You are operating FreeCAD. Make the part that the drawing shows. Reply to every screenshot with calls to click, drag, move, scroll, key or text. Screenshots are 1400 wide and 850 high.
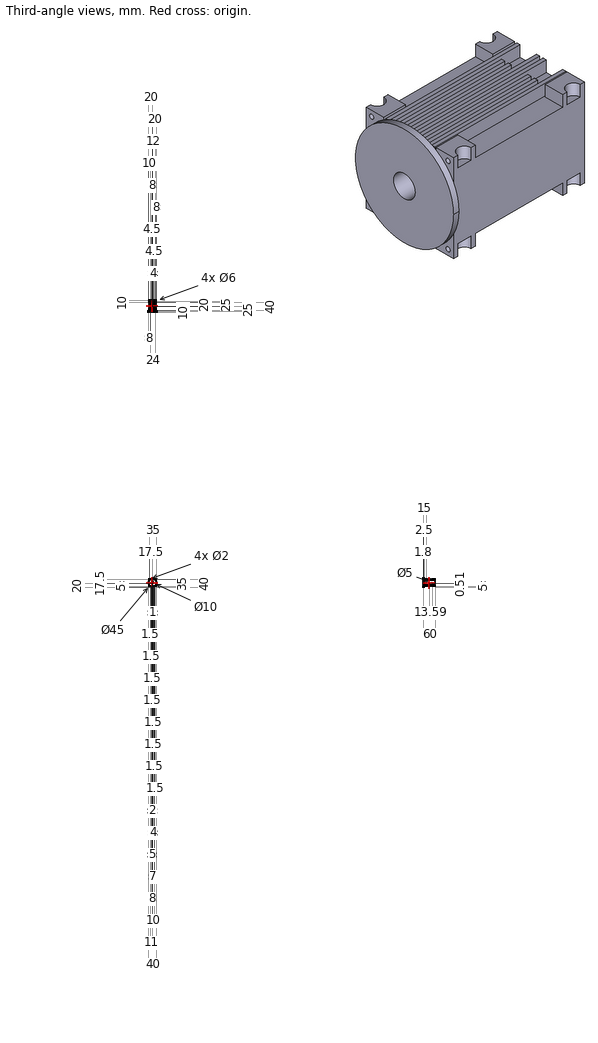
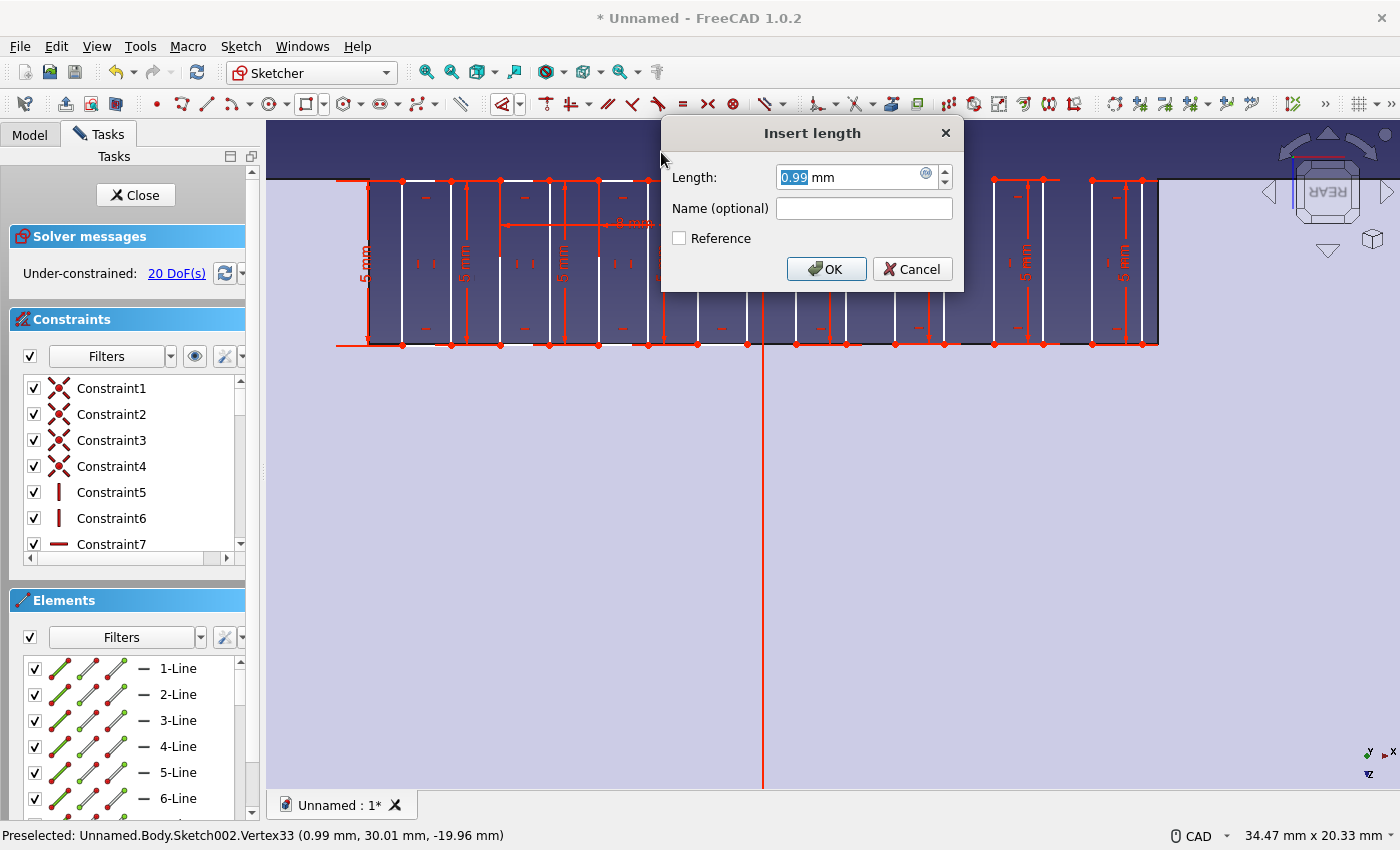
text(1)
key(Return)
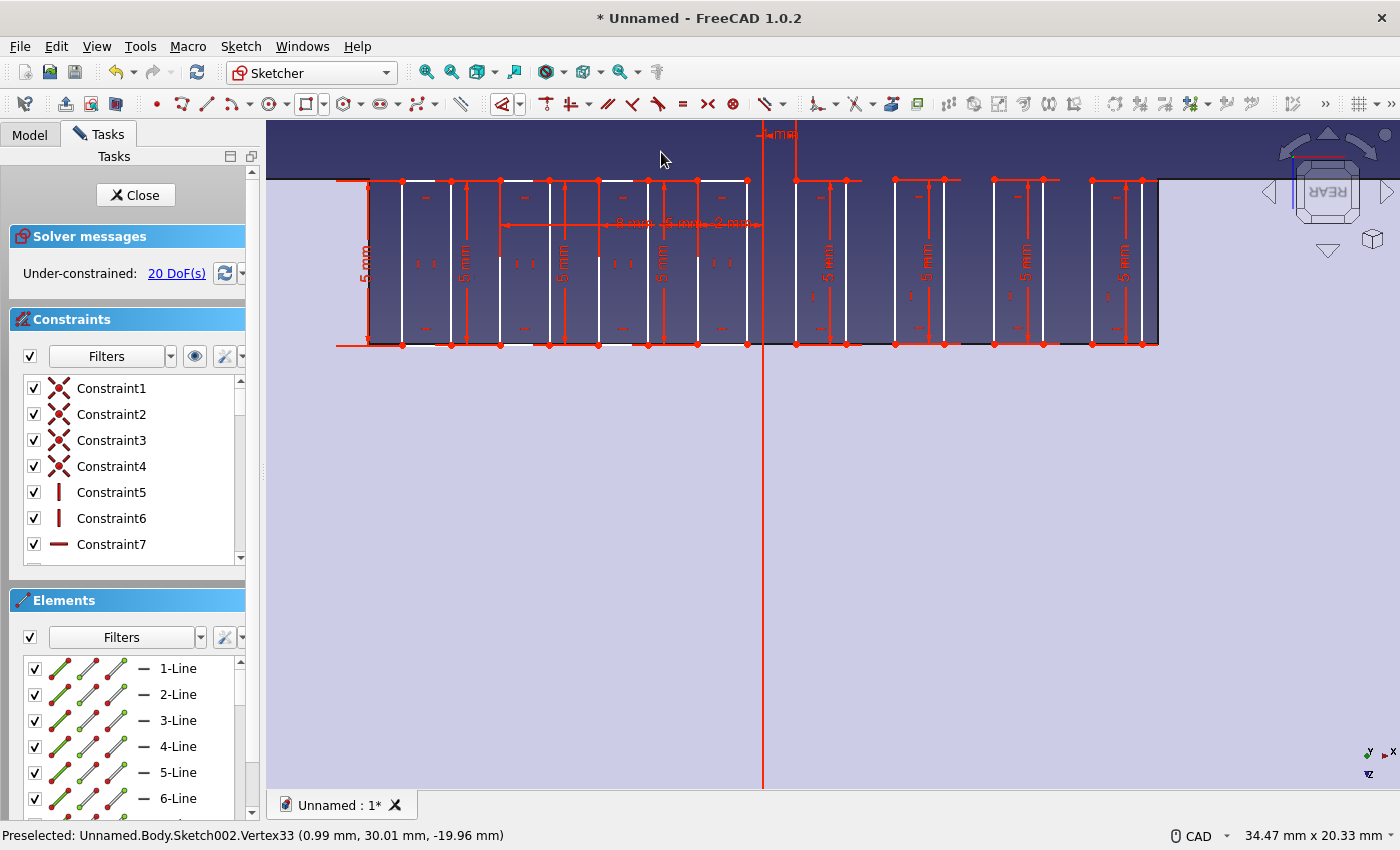
click(895, 180)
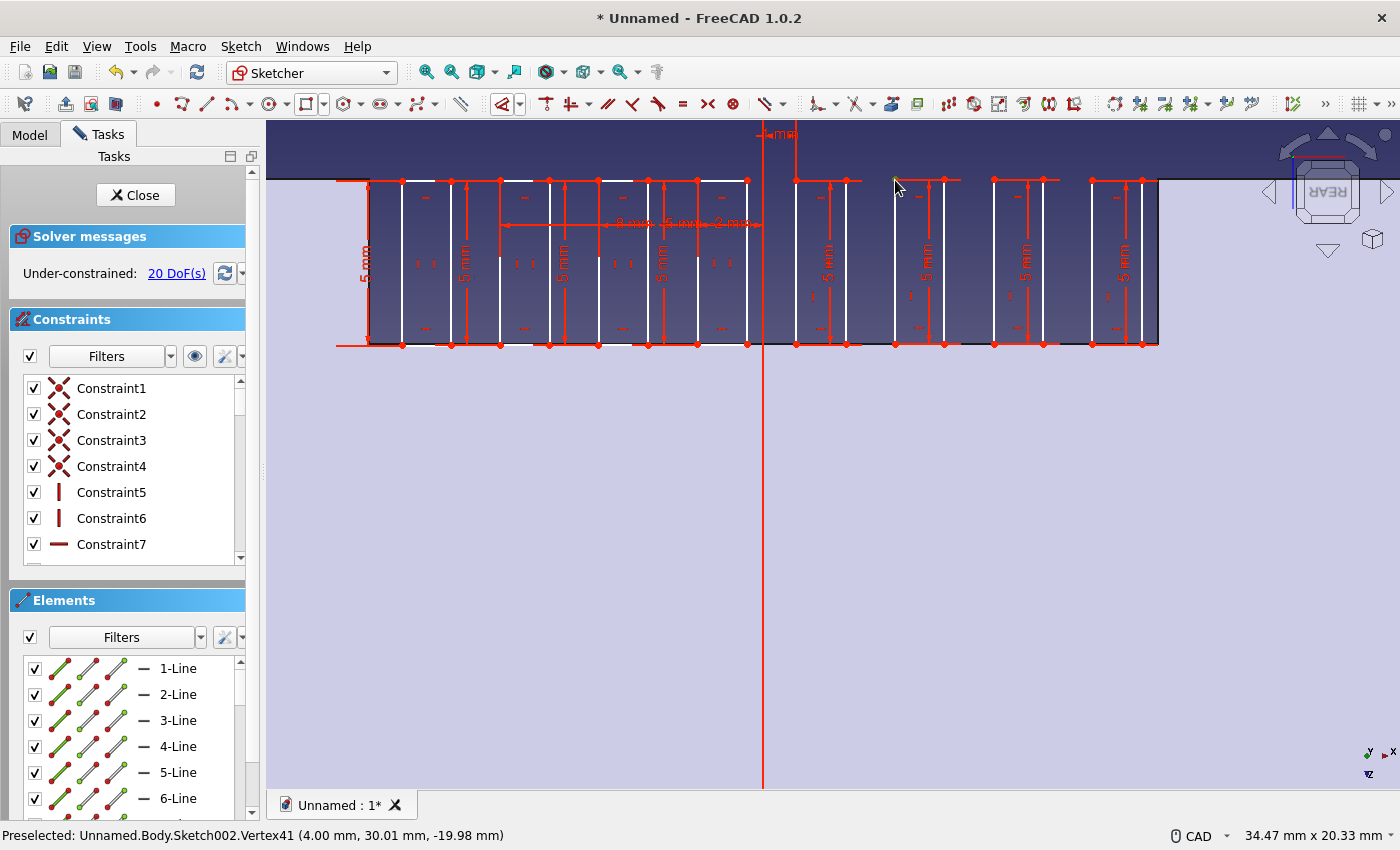
click(520, 104)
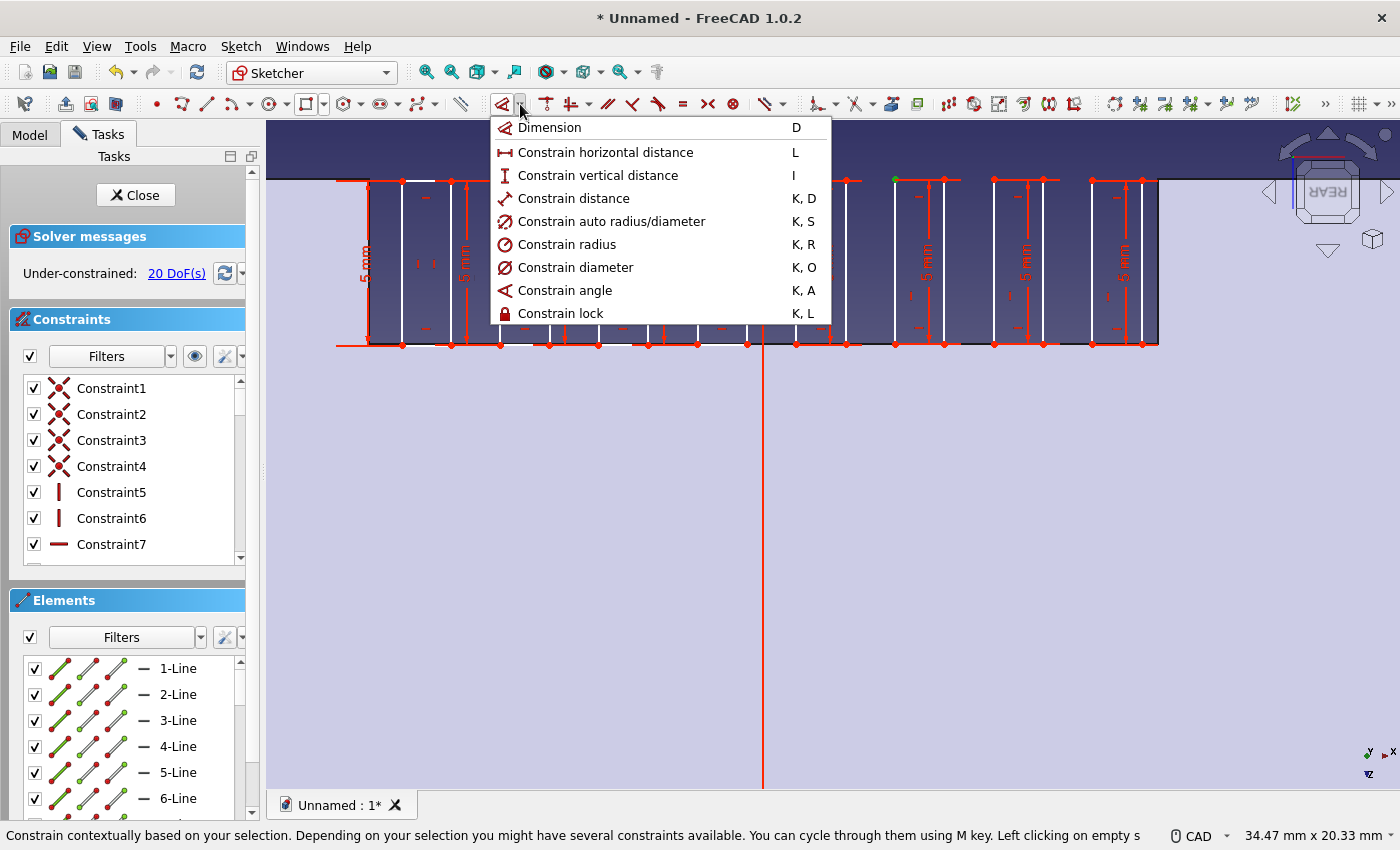
click(661, 152)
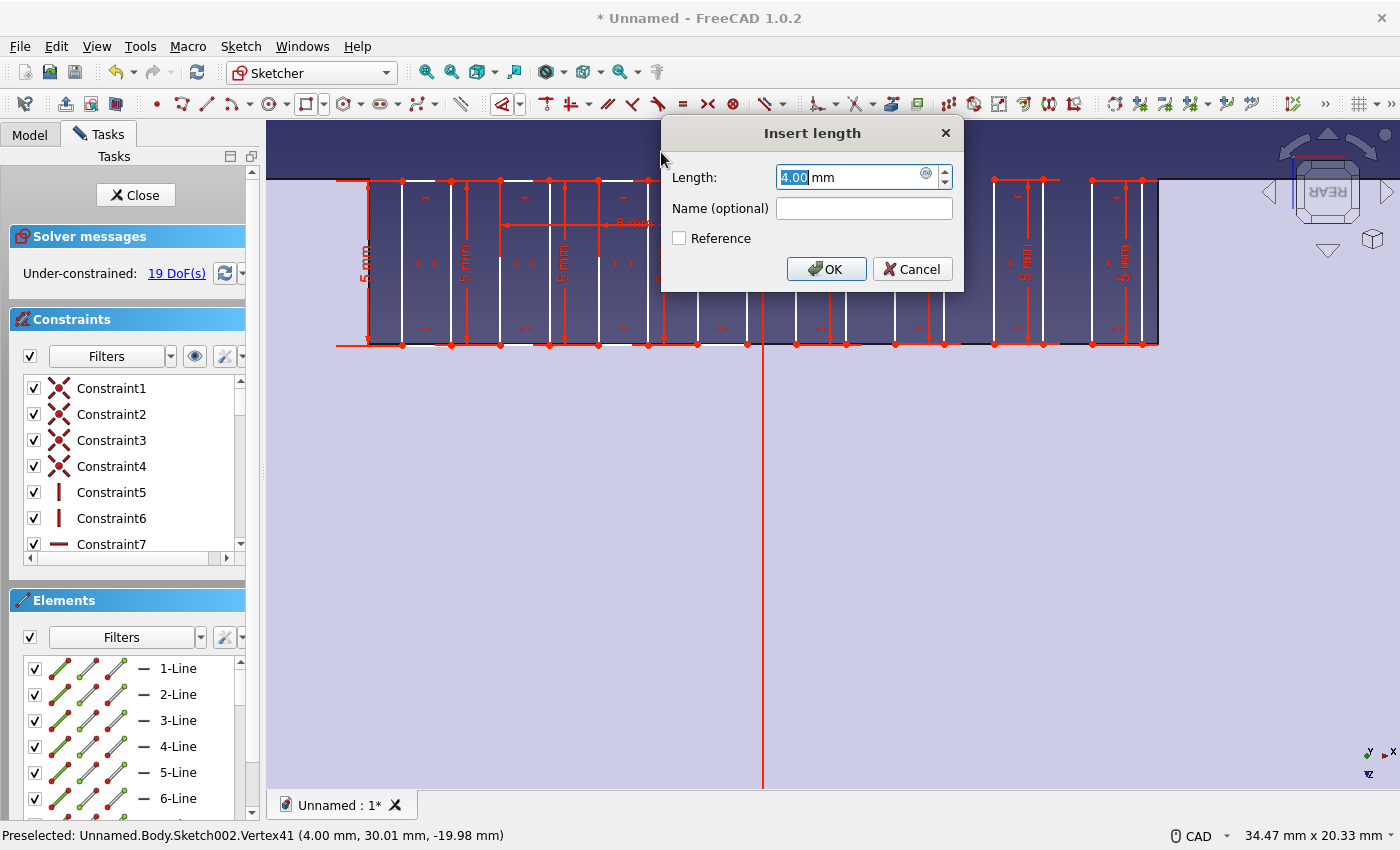
text(4)
key(Return)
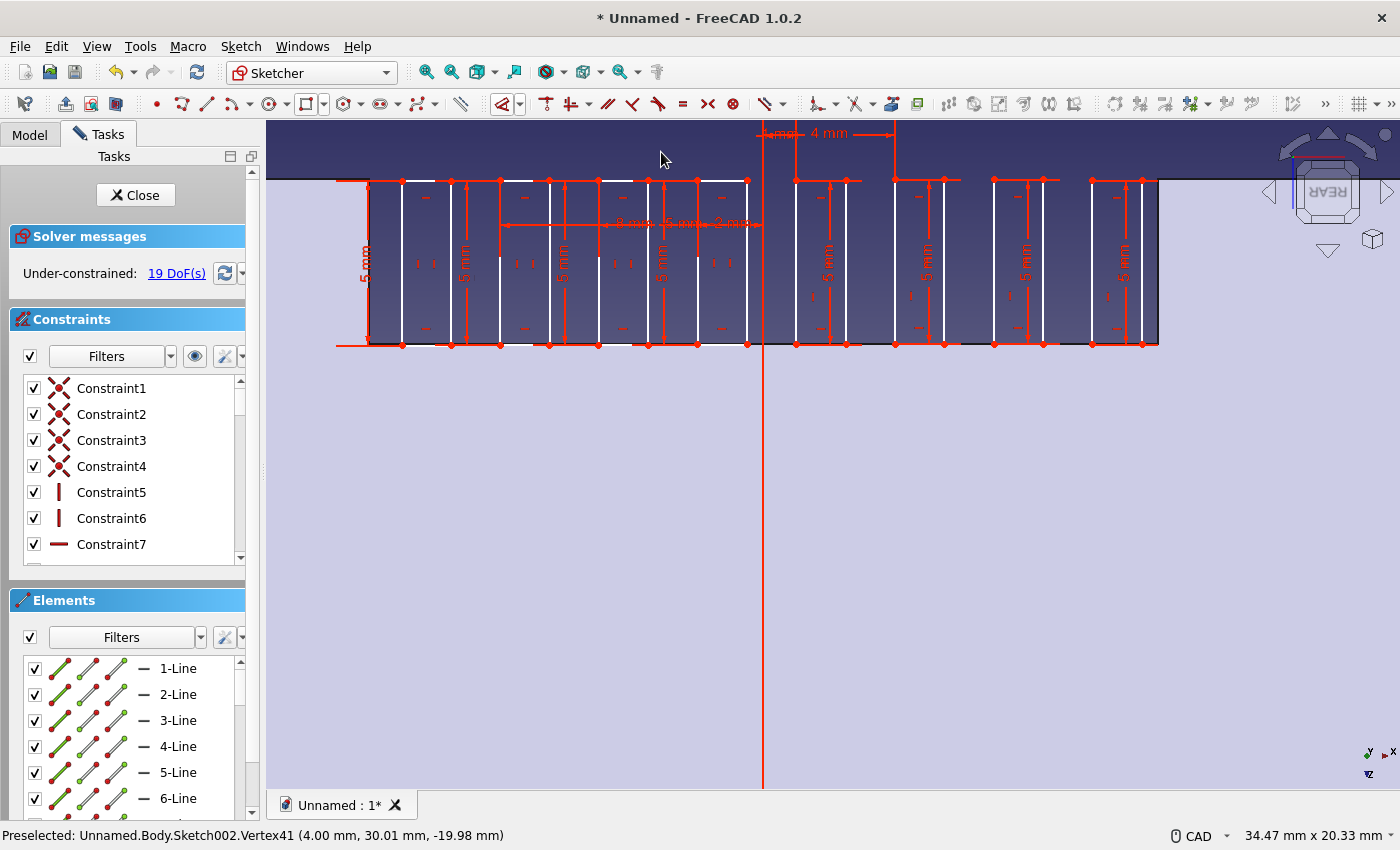
click(994, 180)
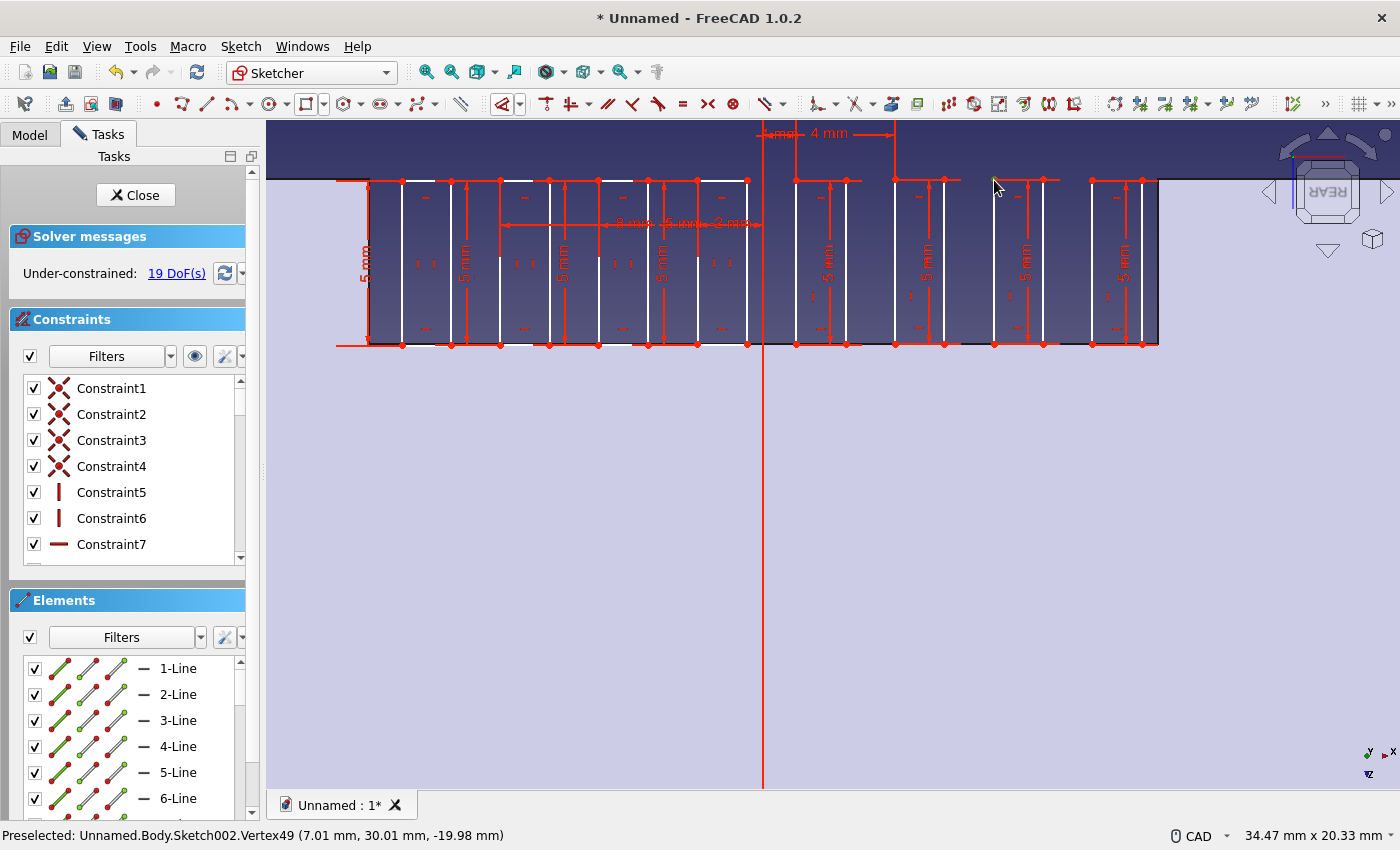
click(520, 104)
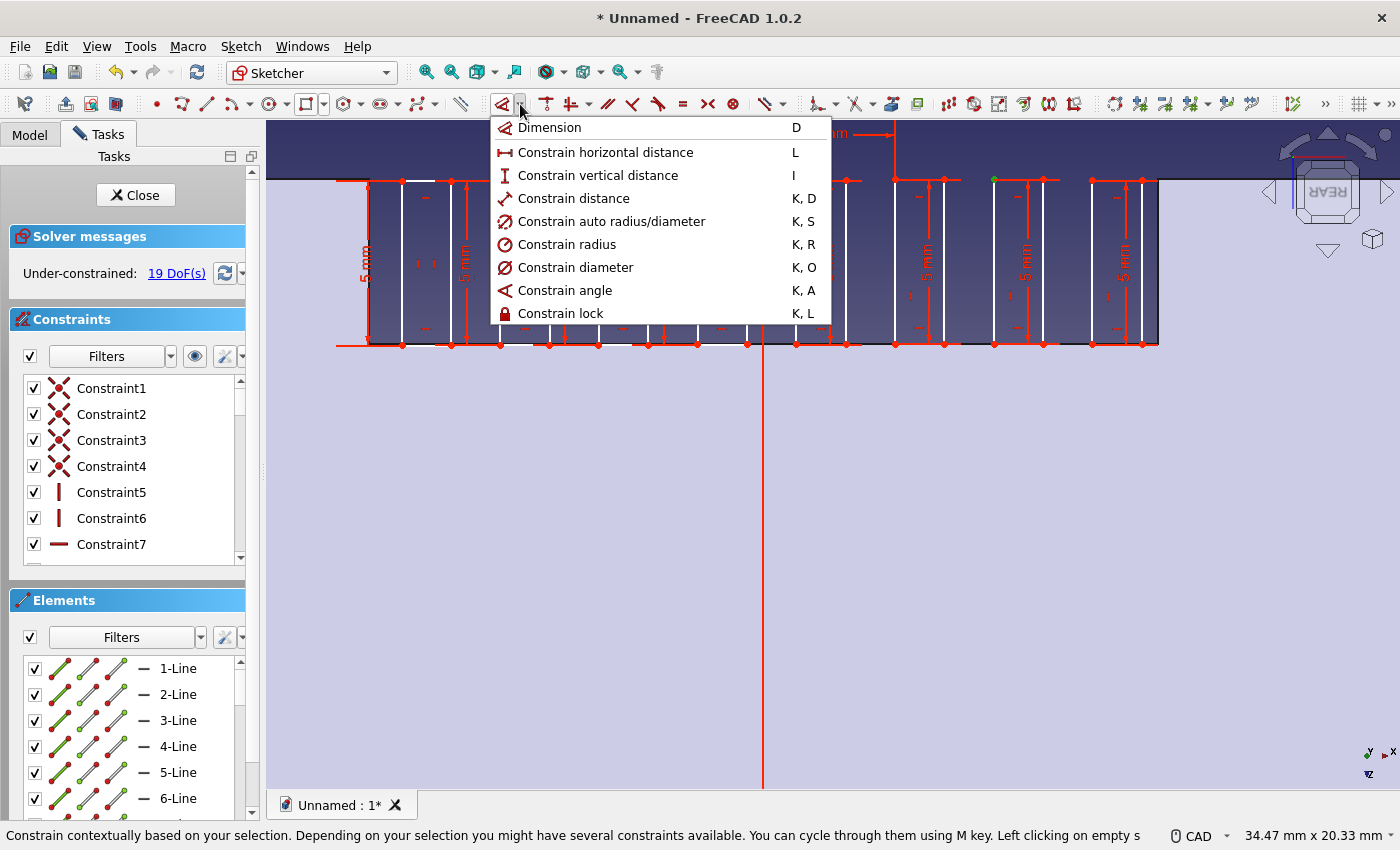
click(661, 152)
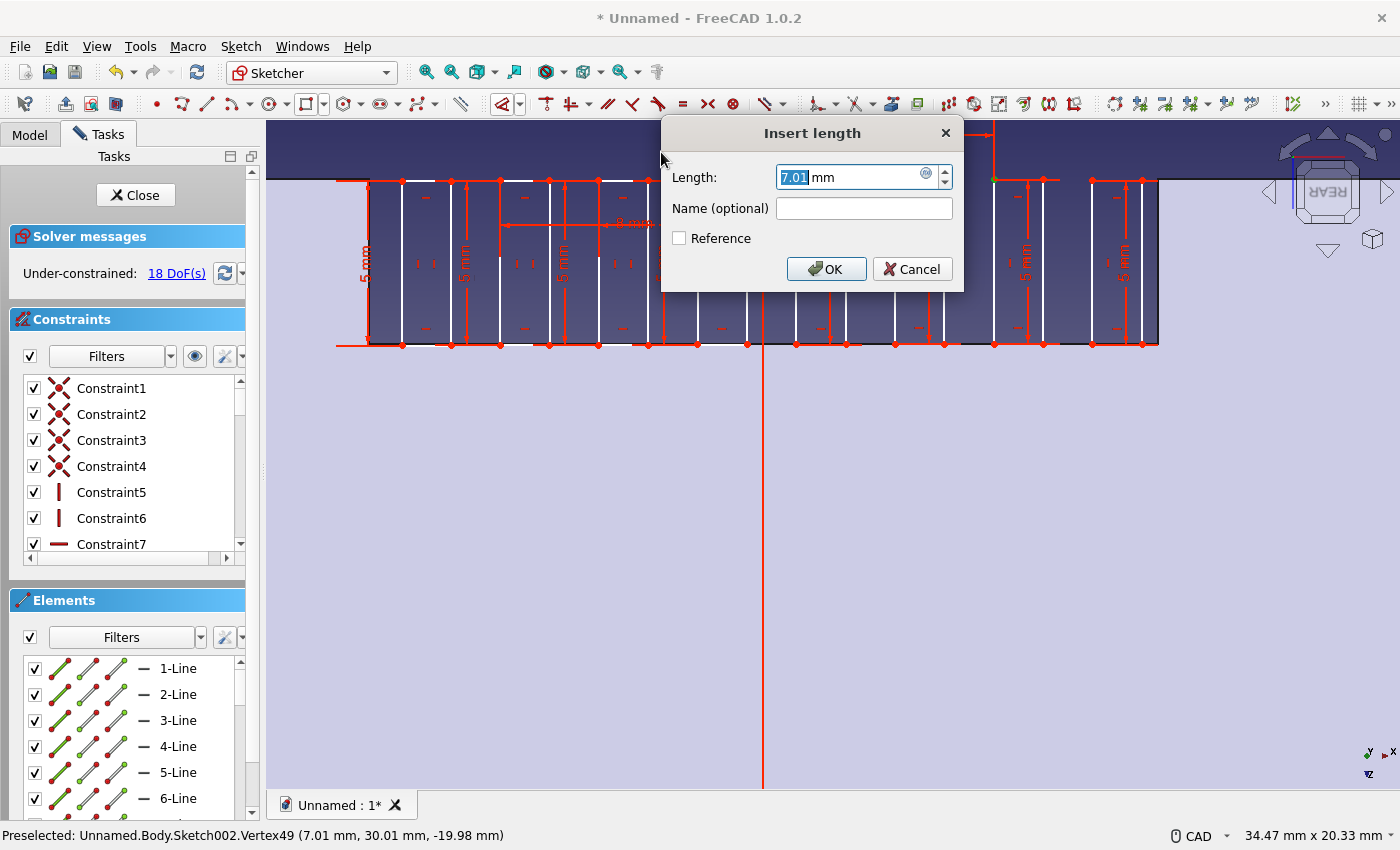
text(7)
key(Return)